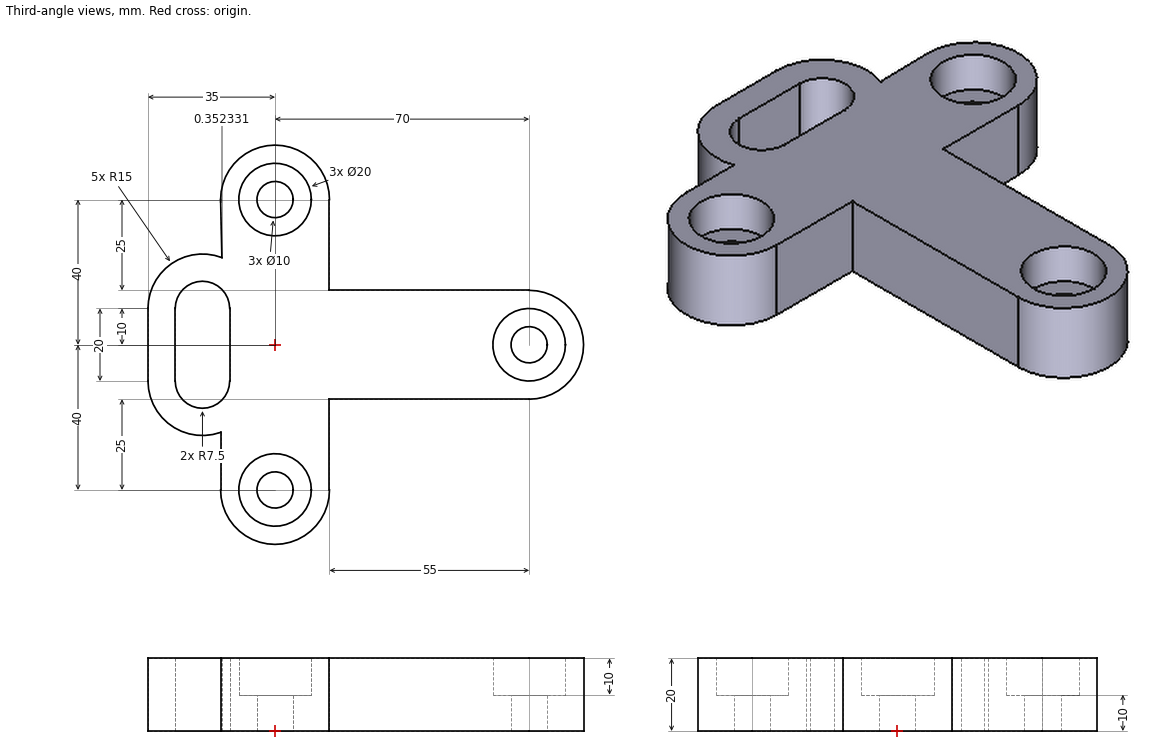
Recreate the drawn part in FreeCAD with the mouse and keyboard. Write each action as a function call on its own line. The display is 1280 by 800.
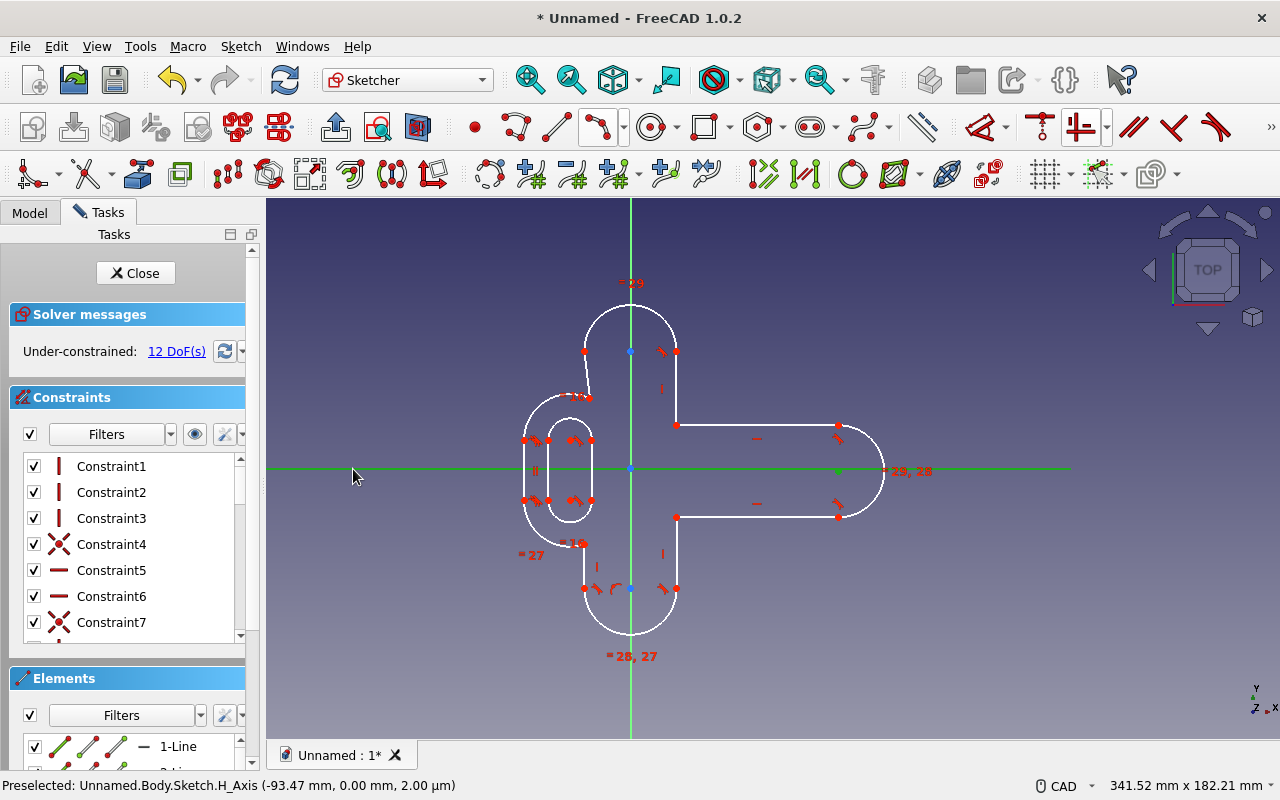
click(1040, 128)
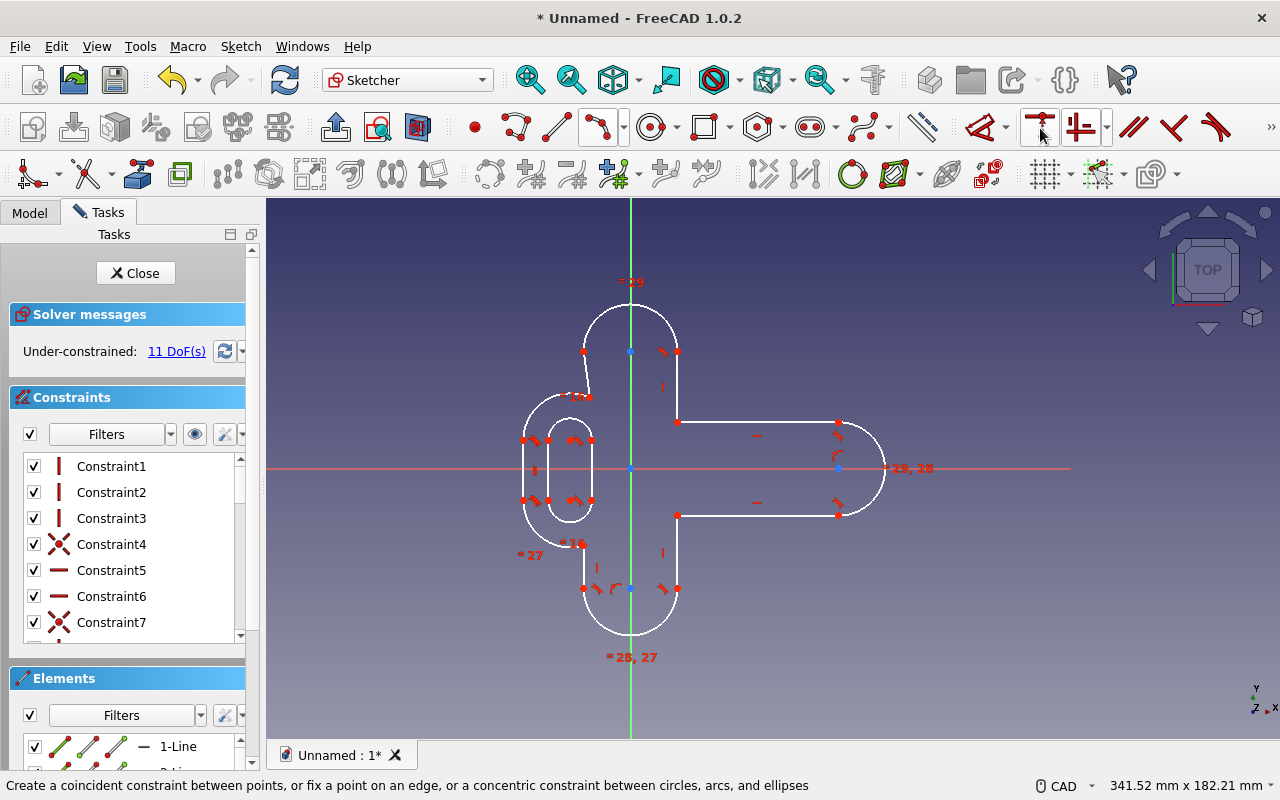
click(630, 351)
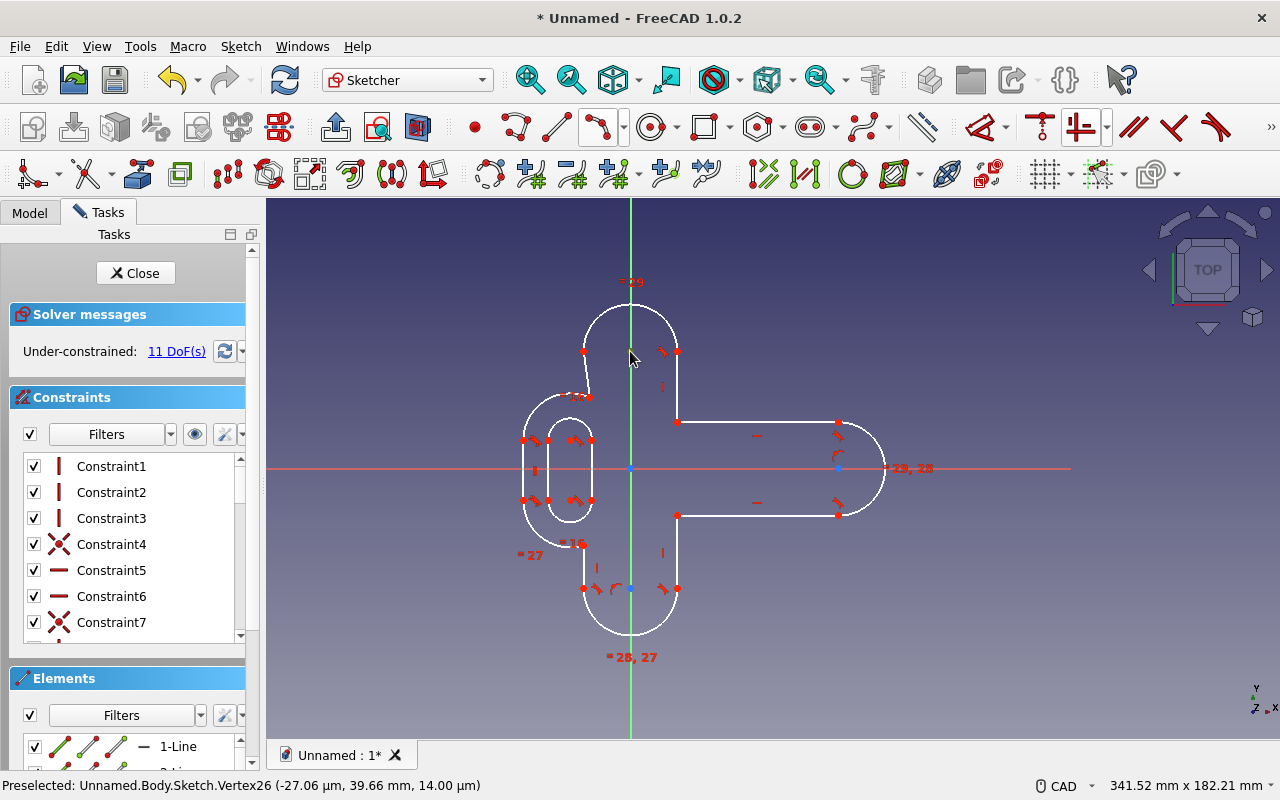
click(631, 676)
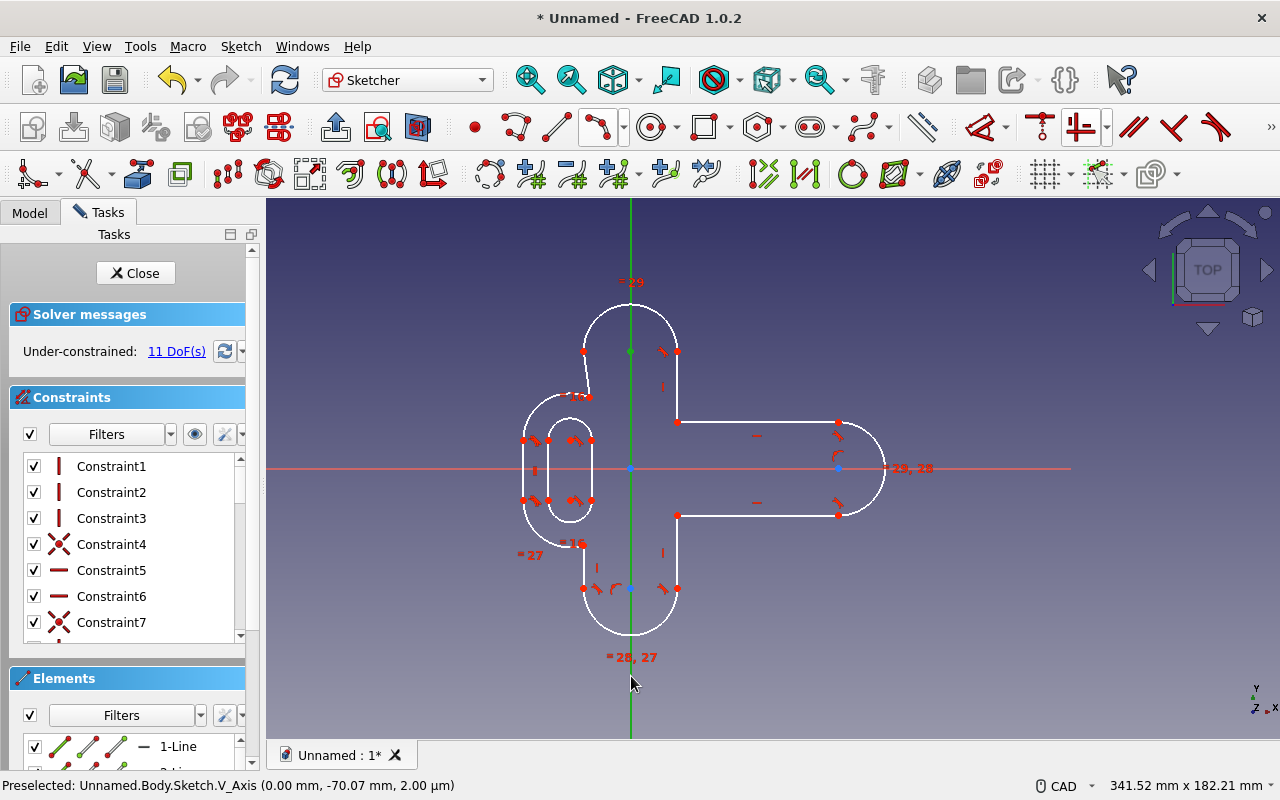
click(1040, 128)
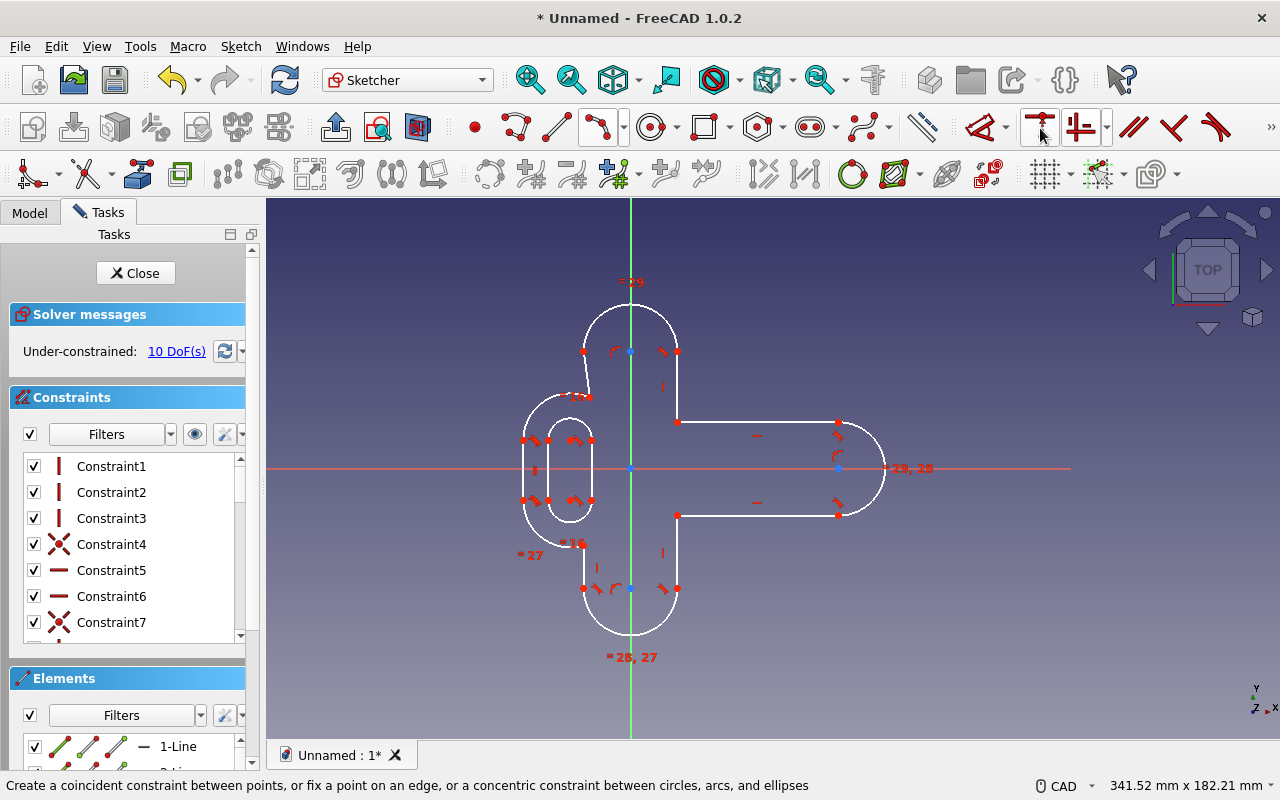
key(d)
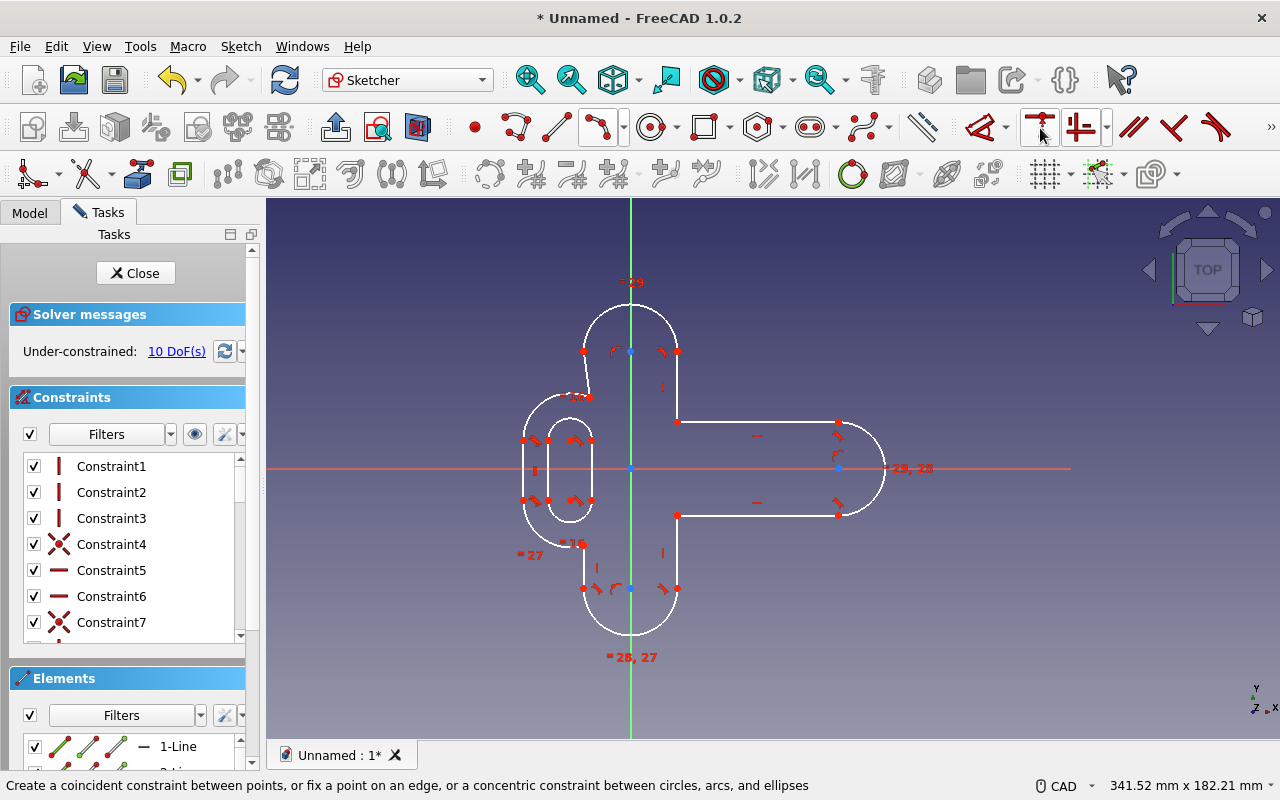
click(531, 525)
click(504, 542)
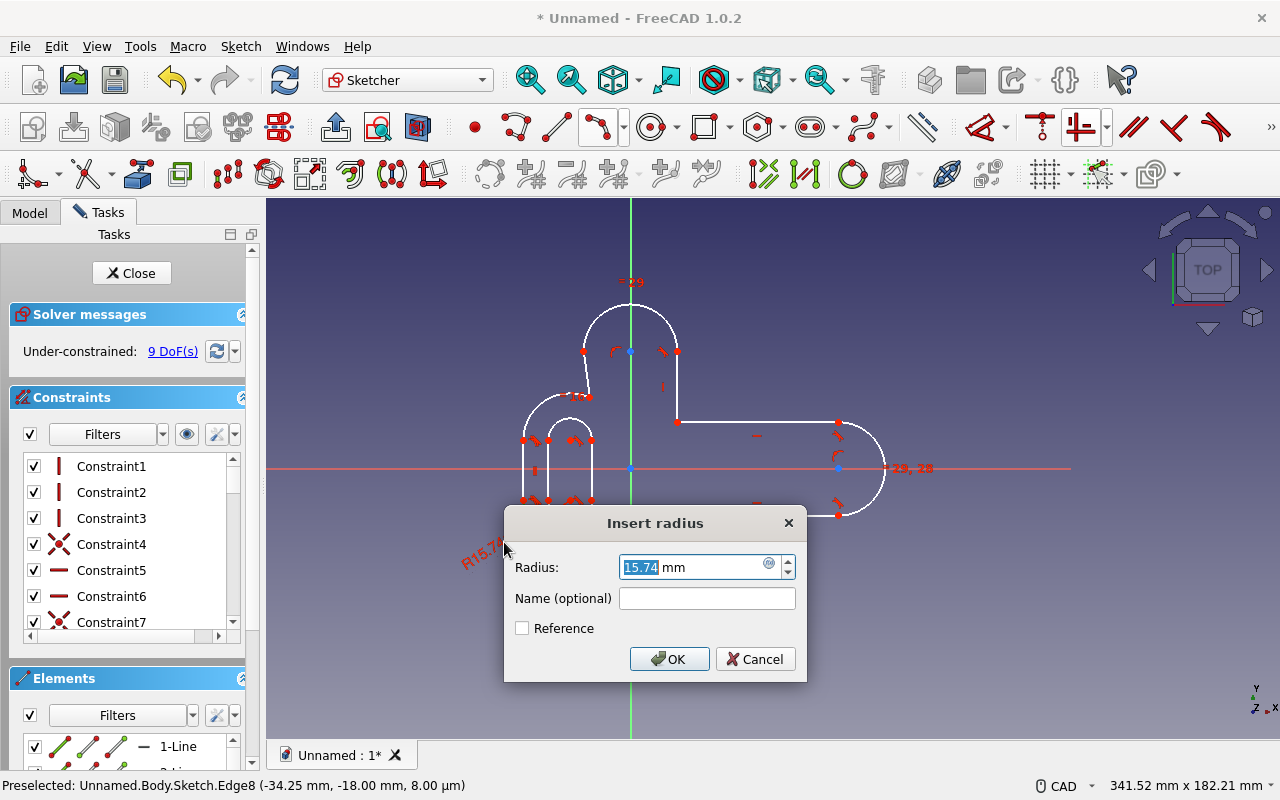
text(15)
key(Return)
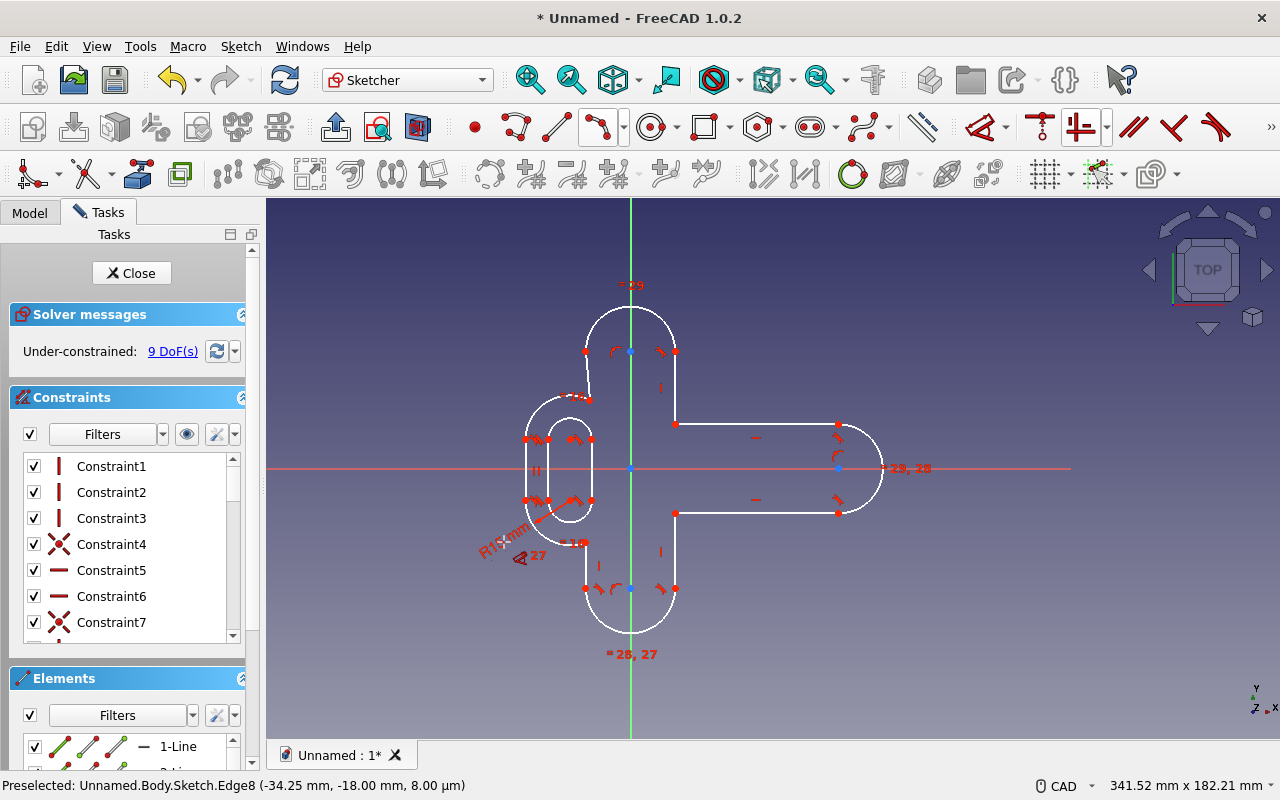
scroll(557, 518, up, 3)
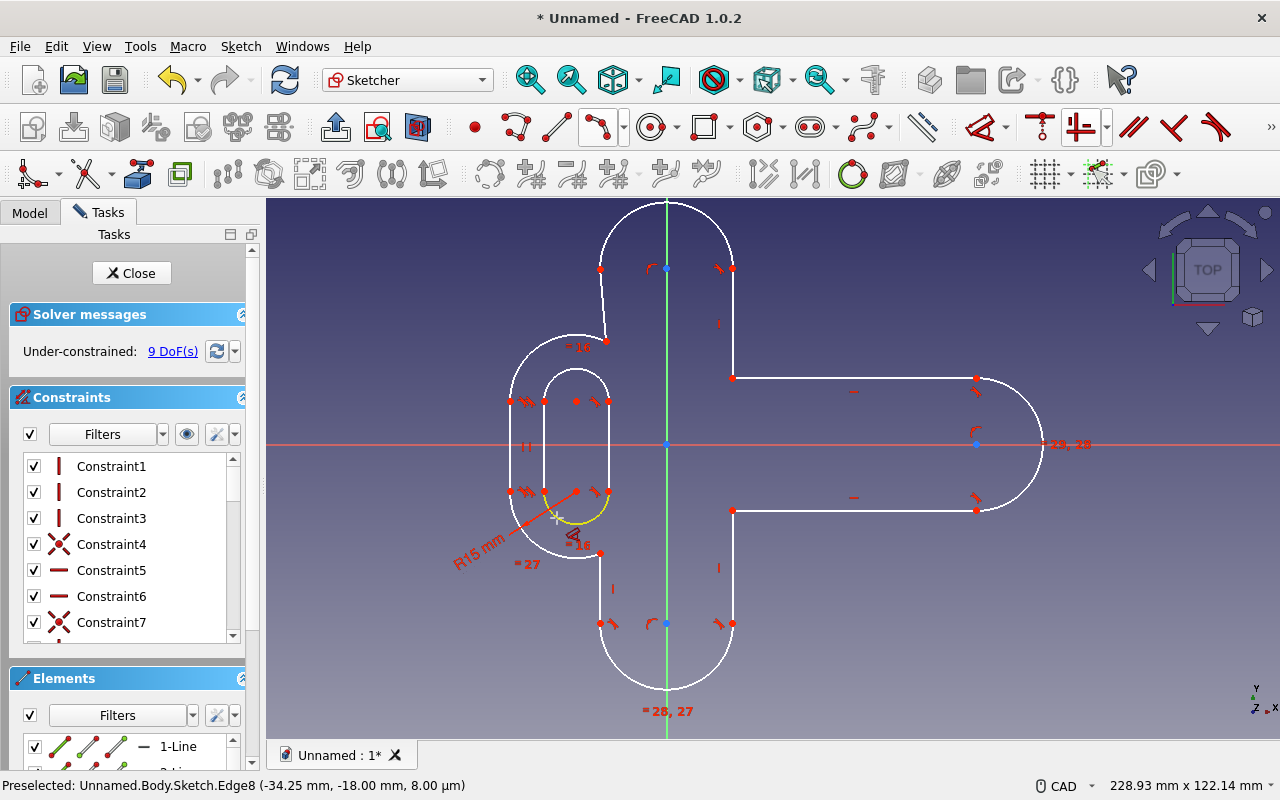
click(557, 518)
click(523, 443)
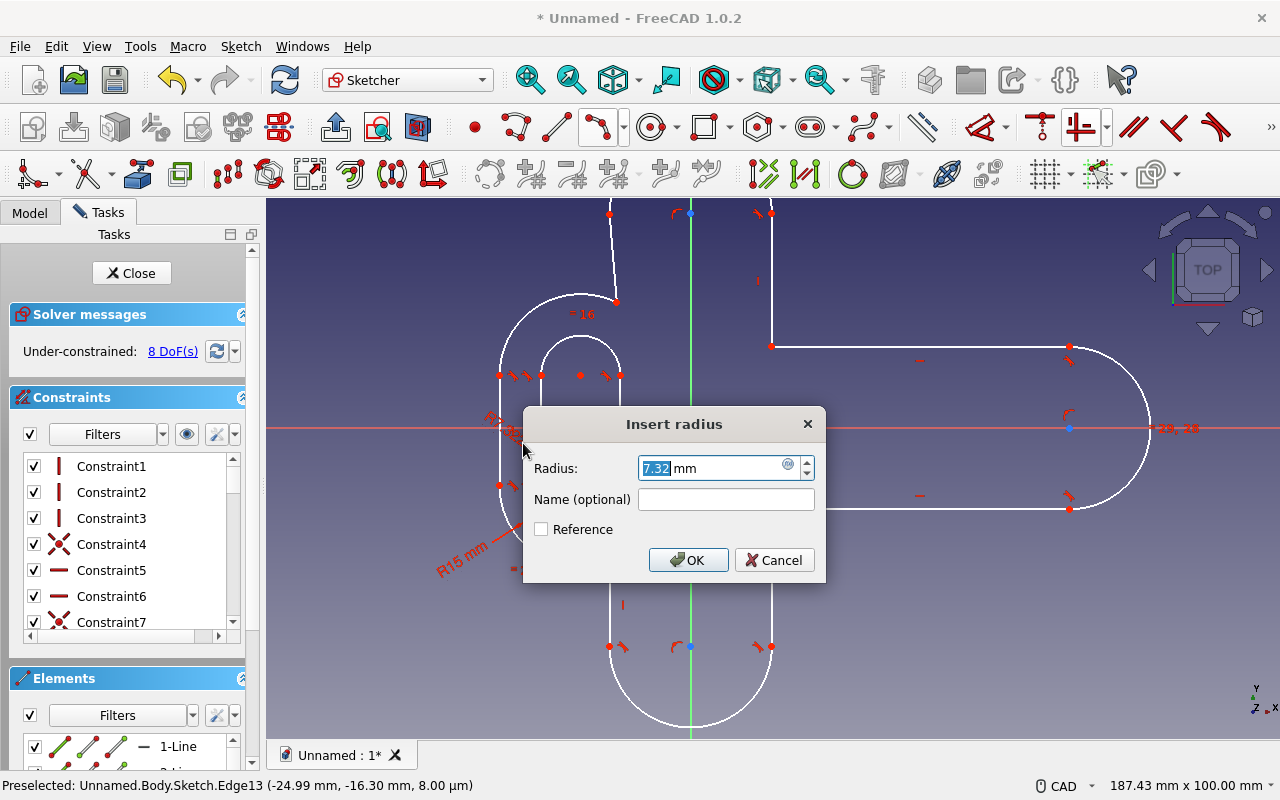
text(7.5)
key(Return)